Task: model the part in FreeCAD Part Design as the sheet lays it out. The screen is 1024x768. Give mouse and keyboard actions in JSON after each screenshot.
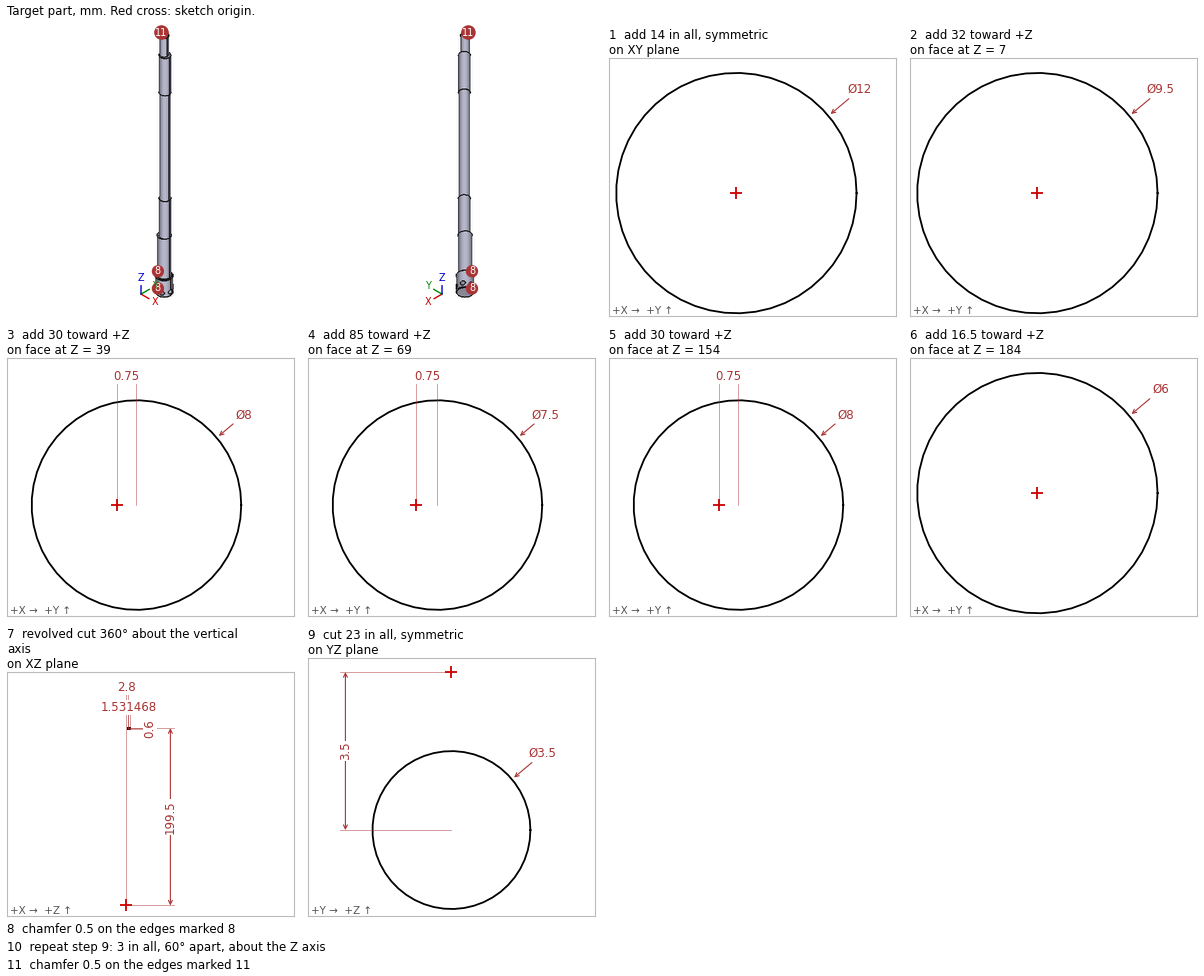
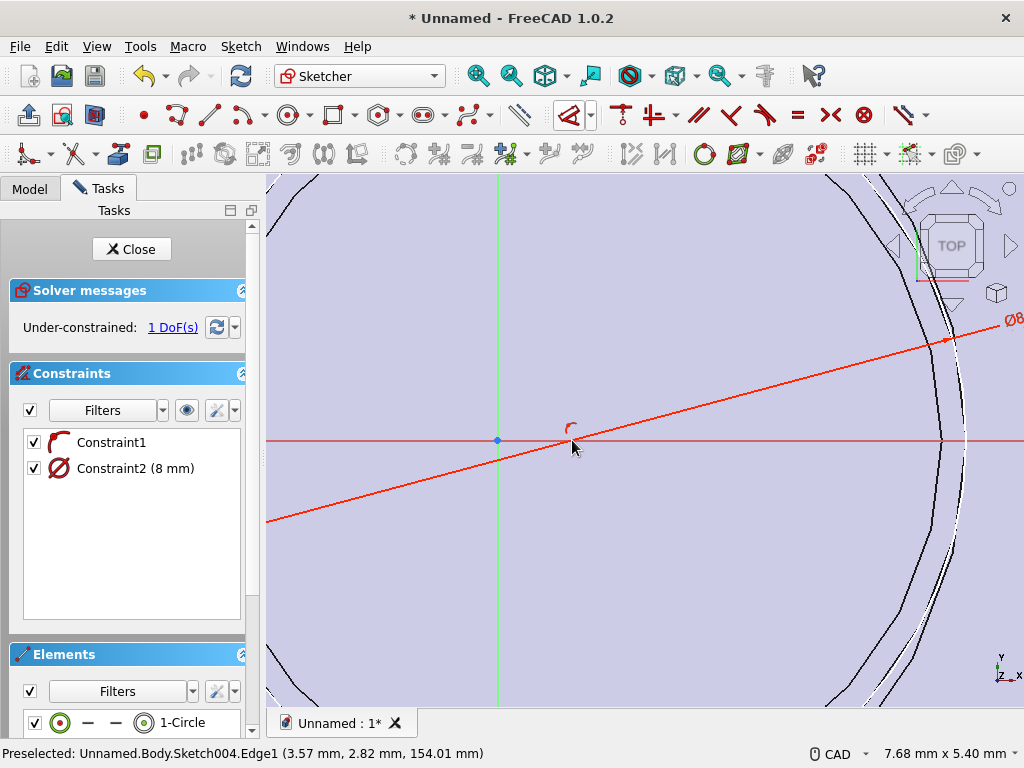
{"action": "left_click", "coordinate": [572, 440]}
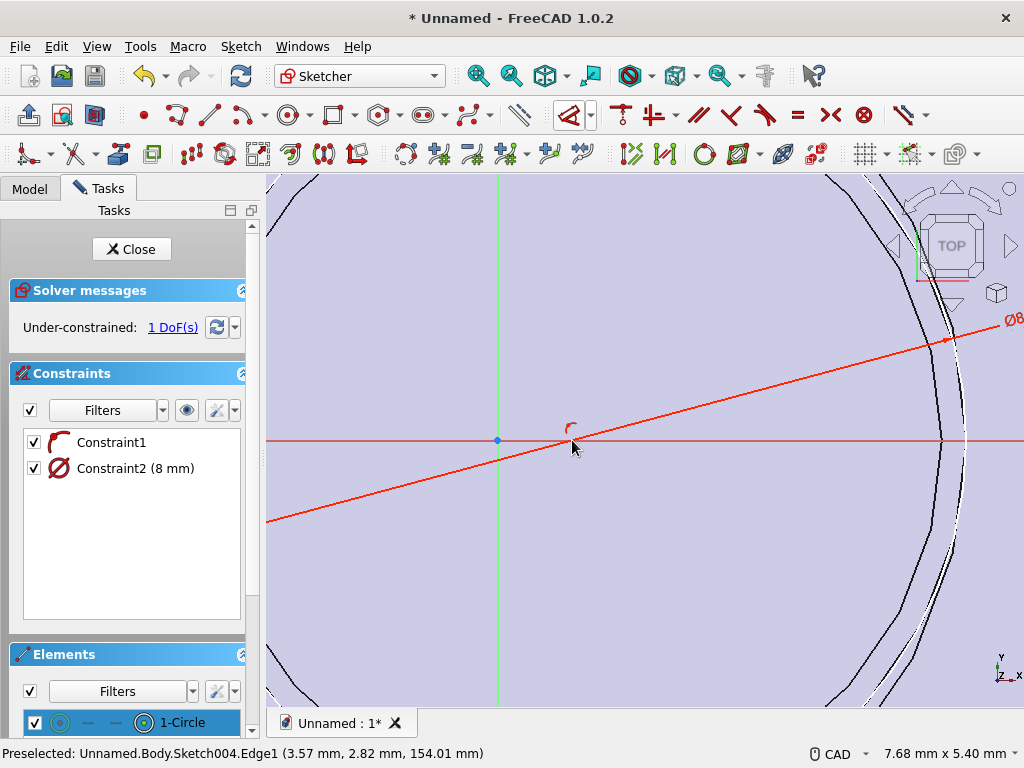
{"action": "key", "text": "l"}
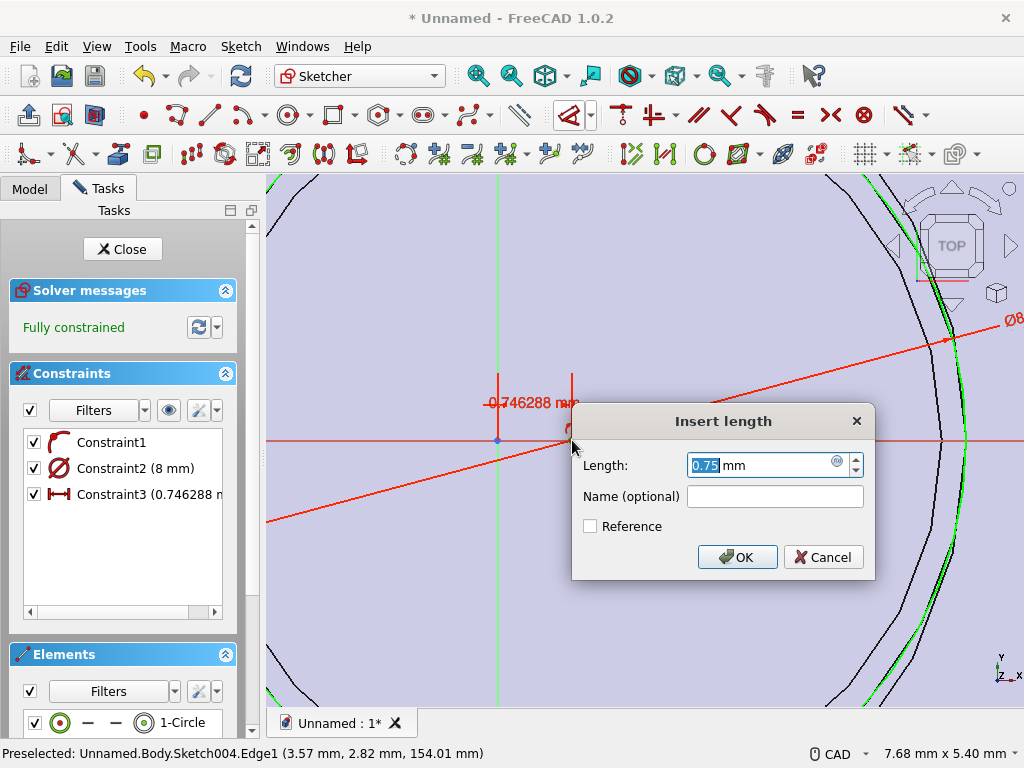
{"action": "type", "text": "0.75"}
{"action": "key", "text": "Return"}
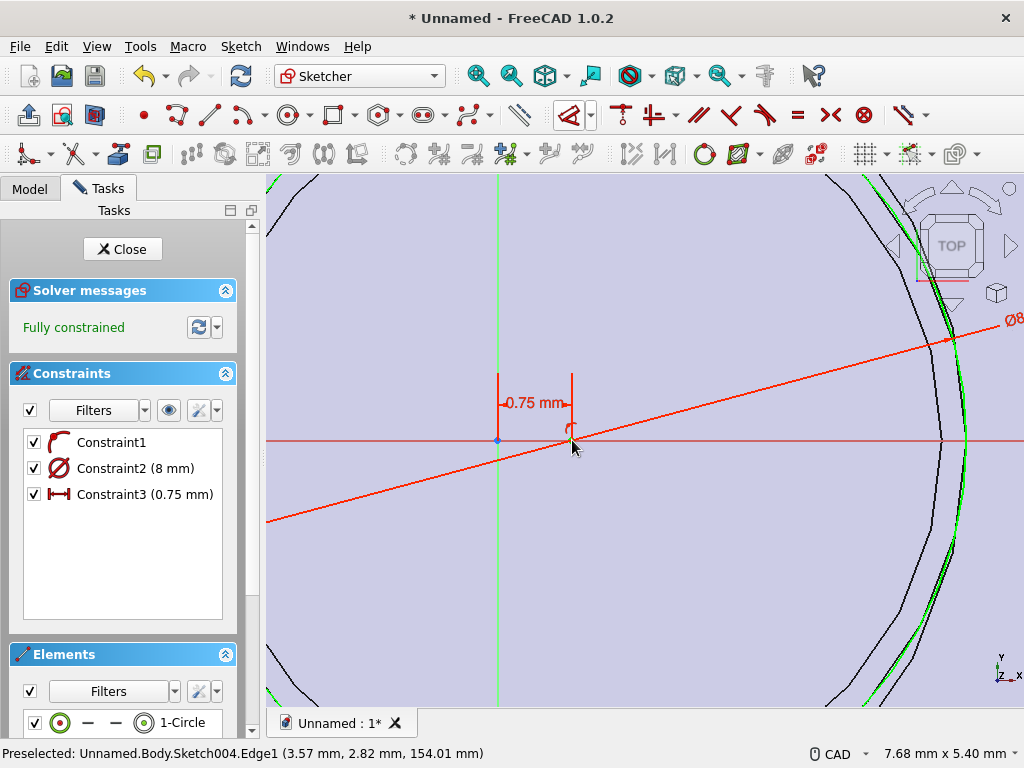
{"action": "left_click", "coordinate": [123, 249]}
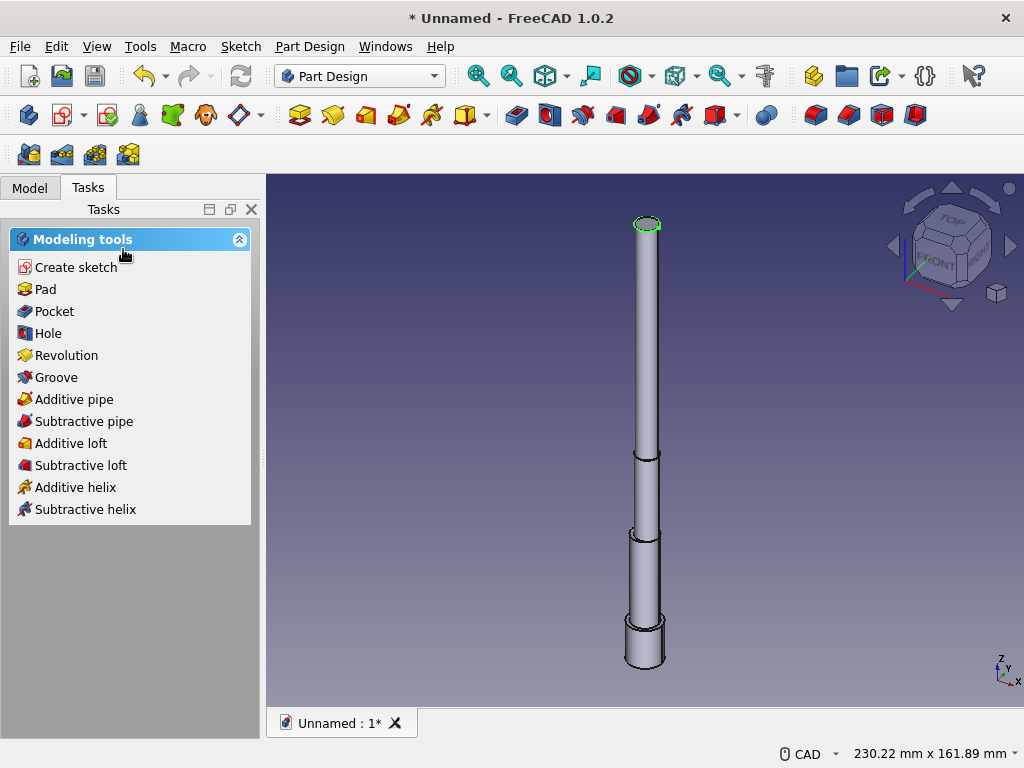
{"action": "left_click", "coordinate": [300, 116]}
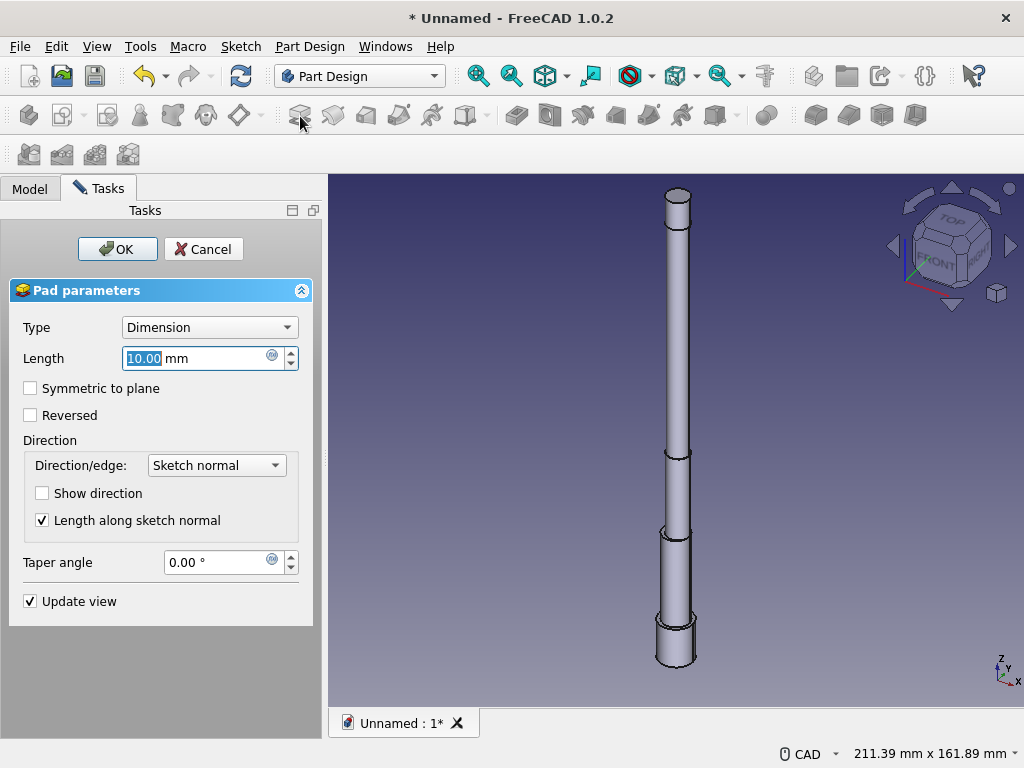
{"action": "type", "text": "30"}
{"action": "key", "text": "Tab"}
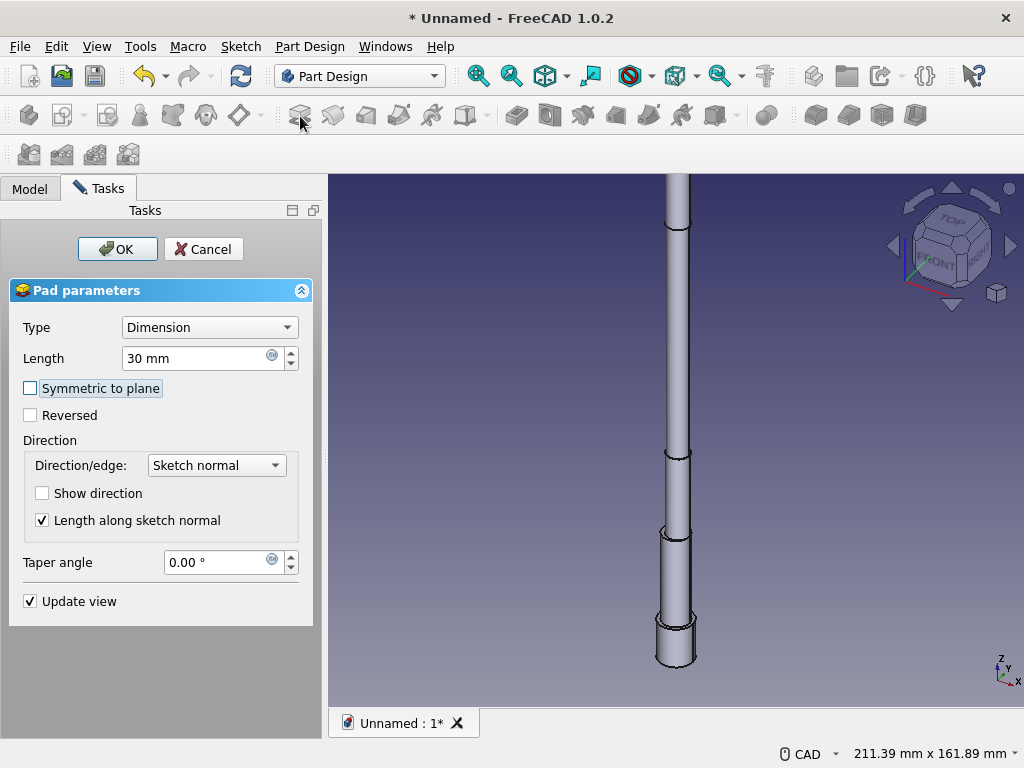
{"action": "left_click", "coordinate": [118, 249]}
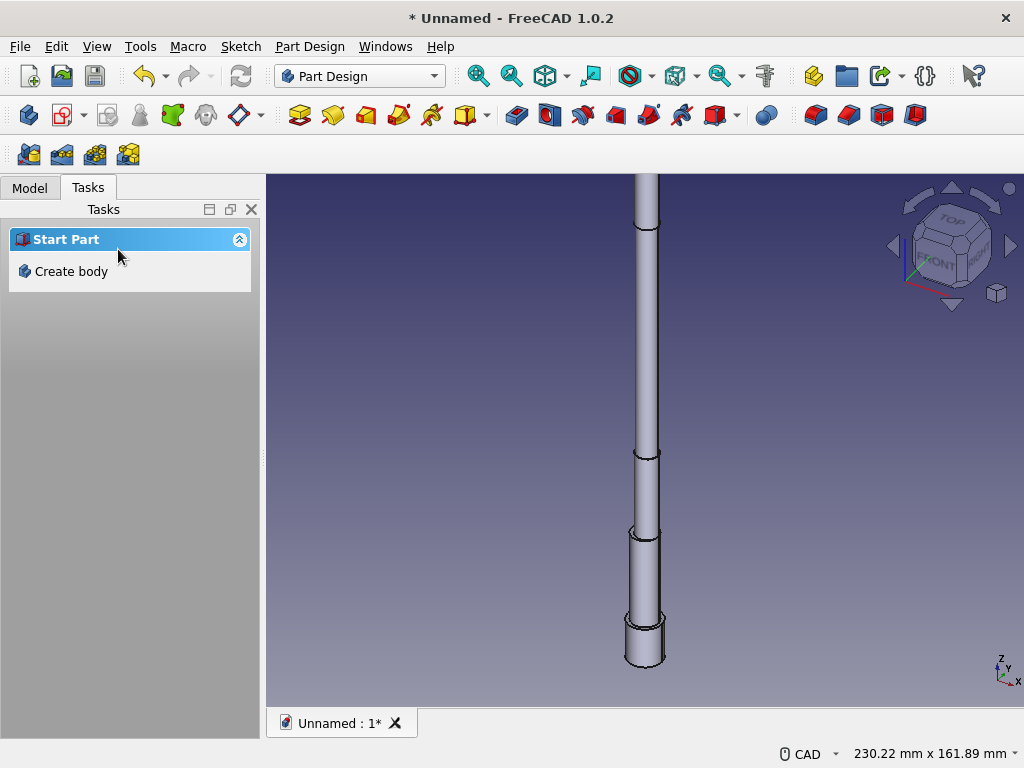
{"action": "key", "text": "v f"}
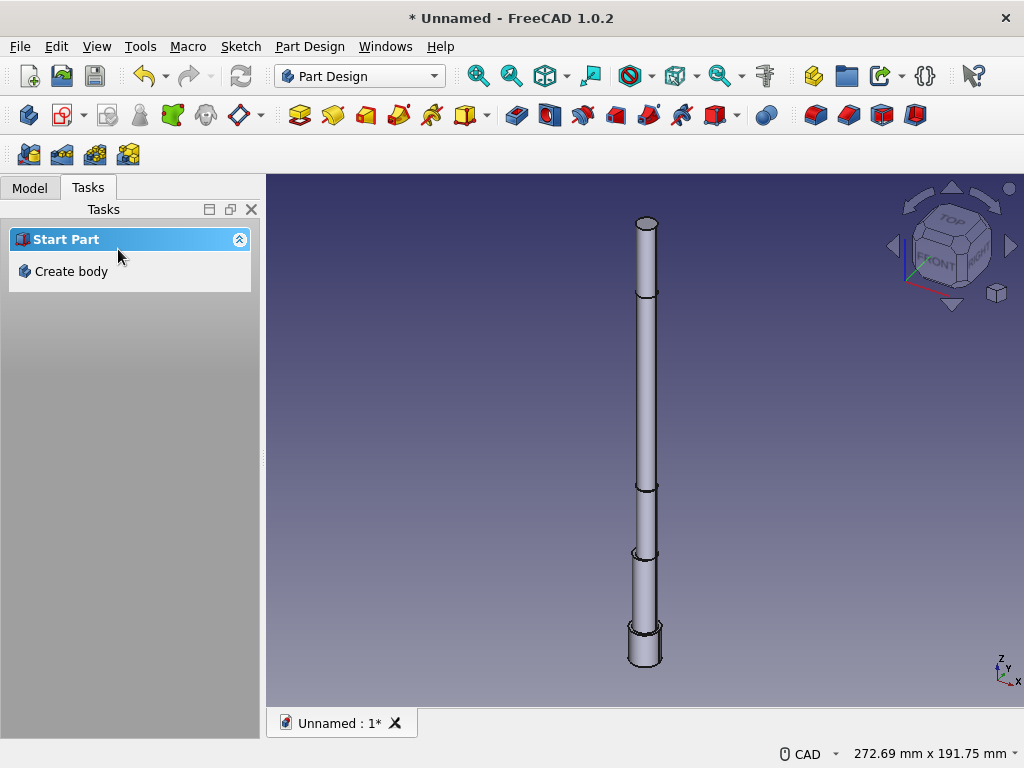
{"action": "key", "text": "0"}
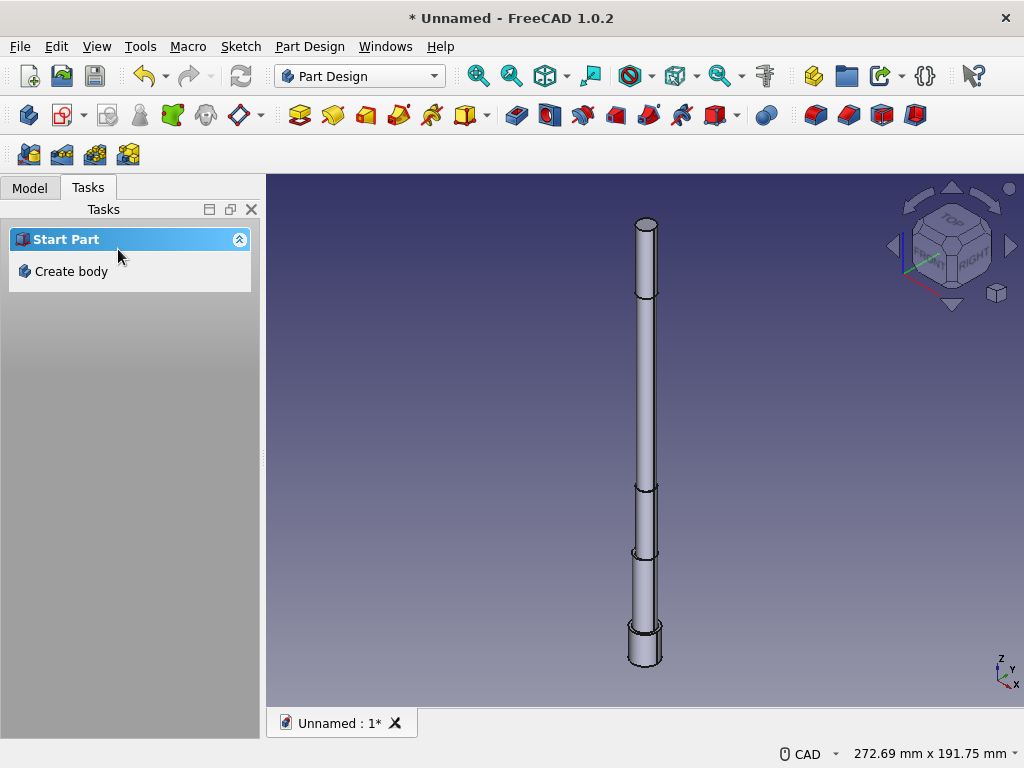
{"action": "key", "text": "2"}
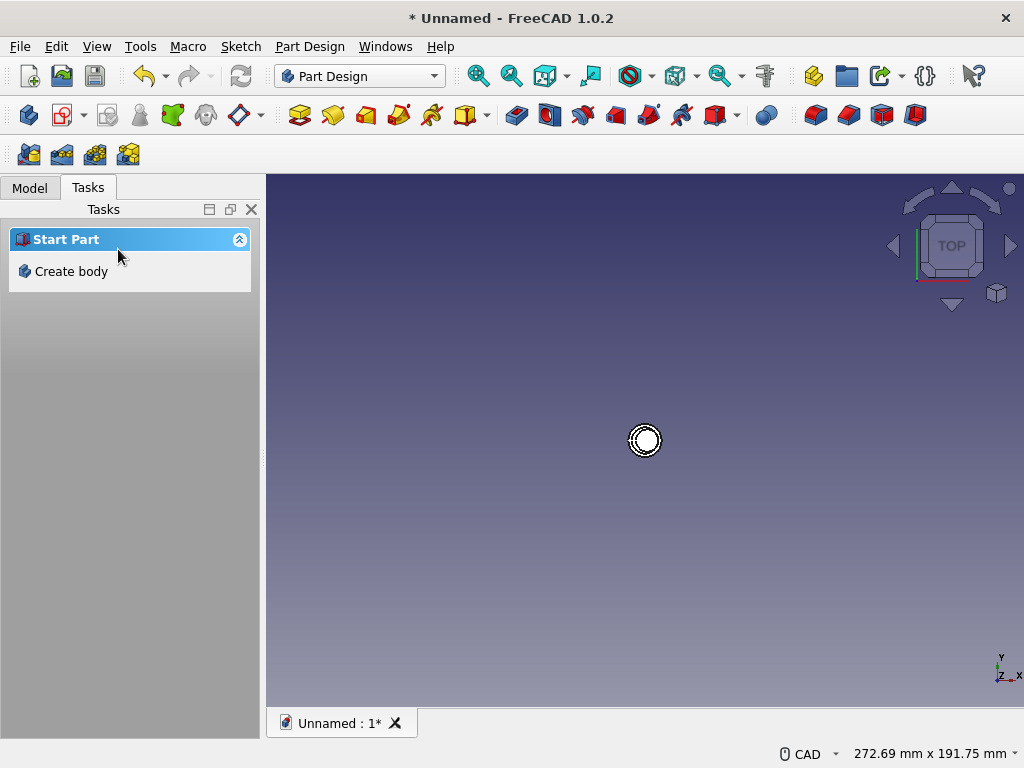
{"action": "key", "text": "v f"}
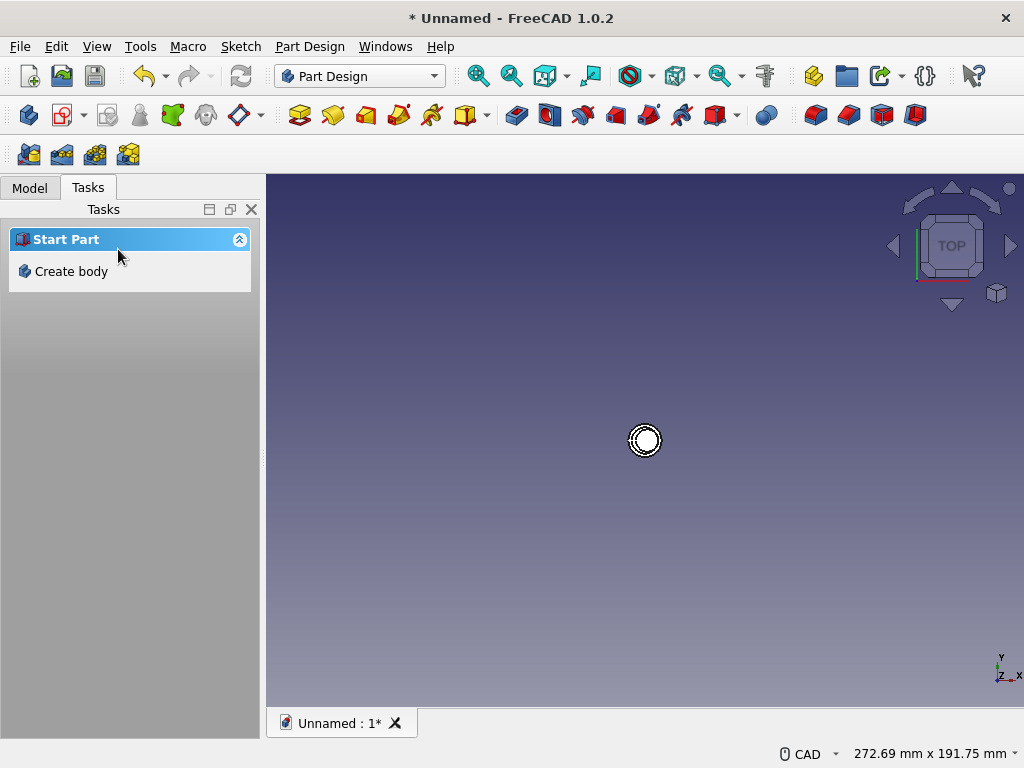
{"action": "left_click", "coordinate": [647, 439]}